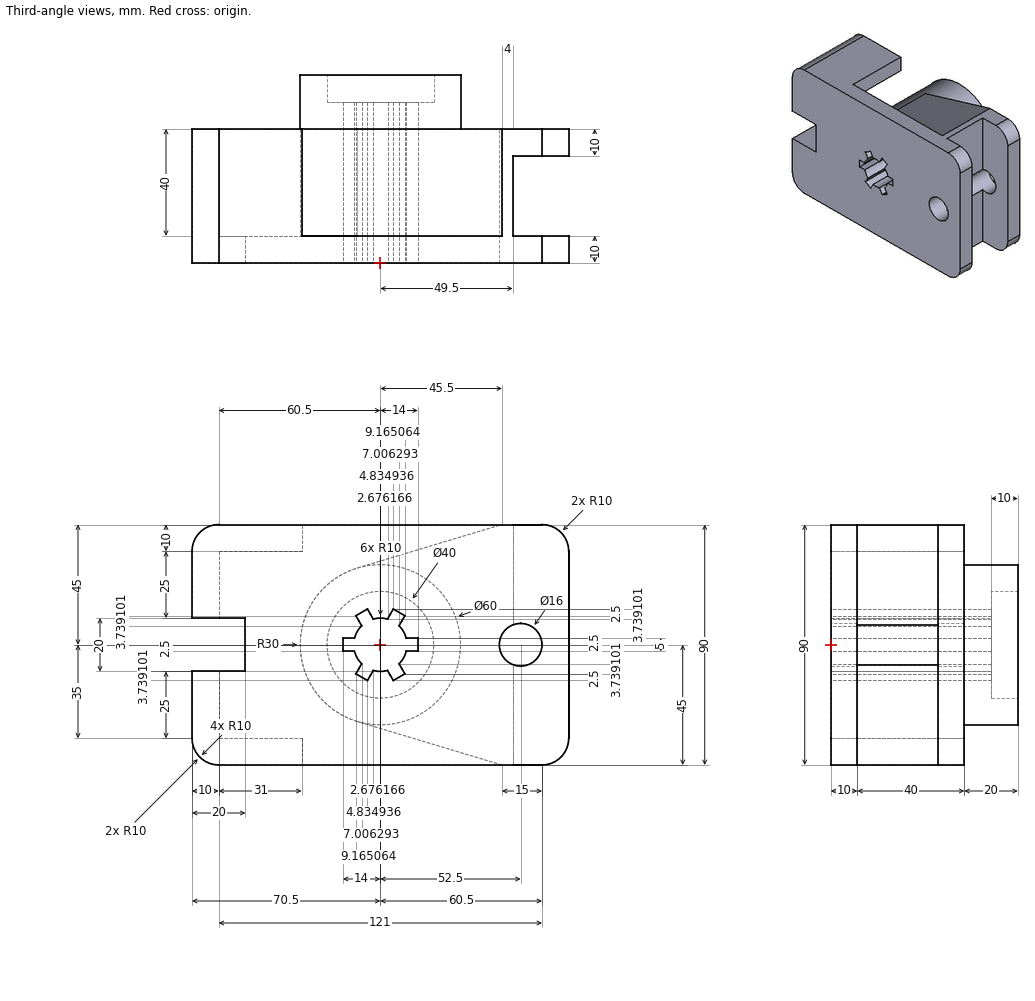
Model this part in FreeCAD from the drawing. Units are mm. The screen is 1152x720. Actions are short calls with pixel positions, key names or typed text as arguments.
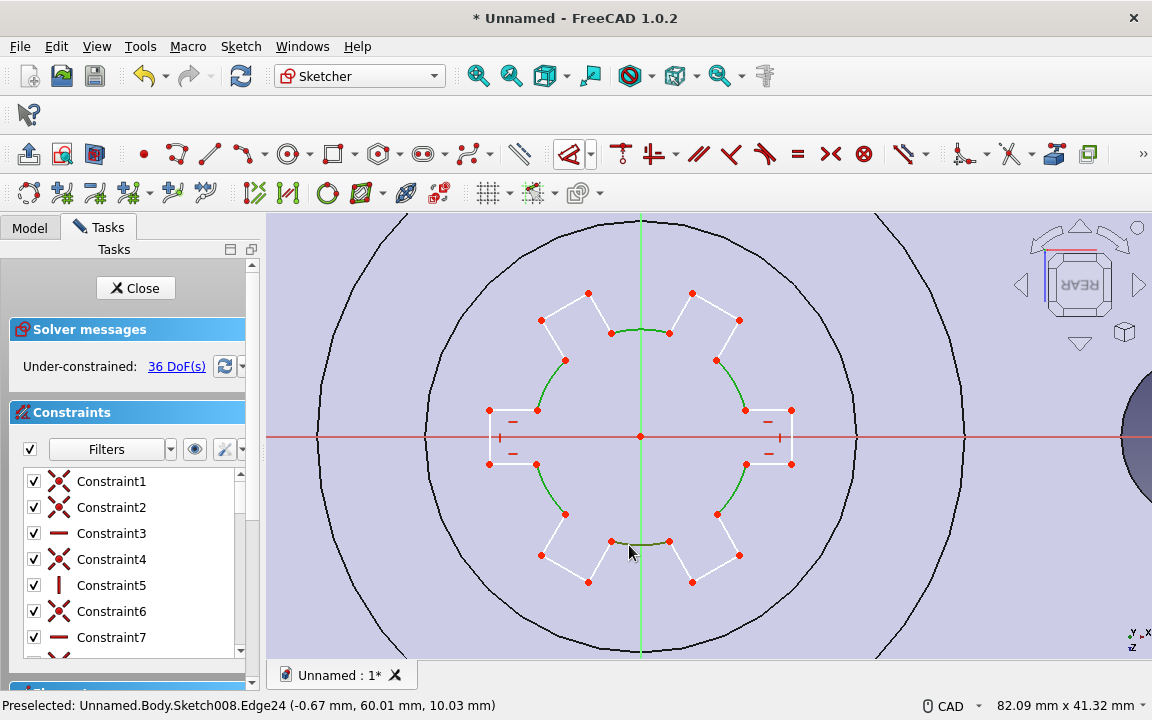
click(798, 154)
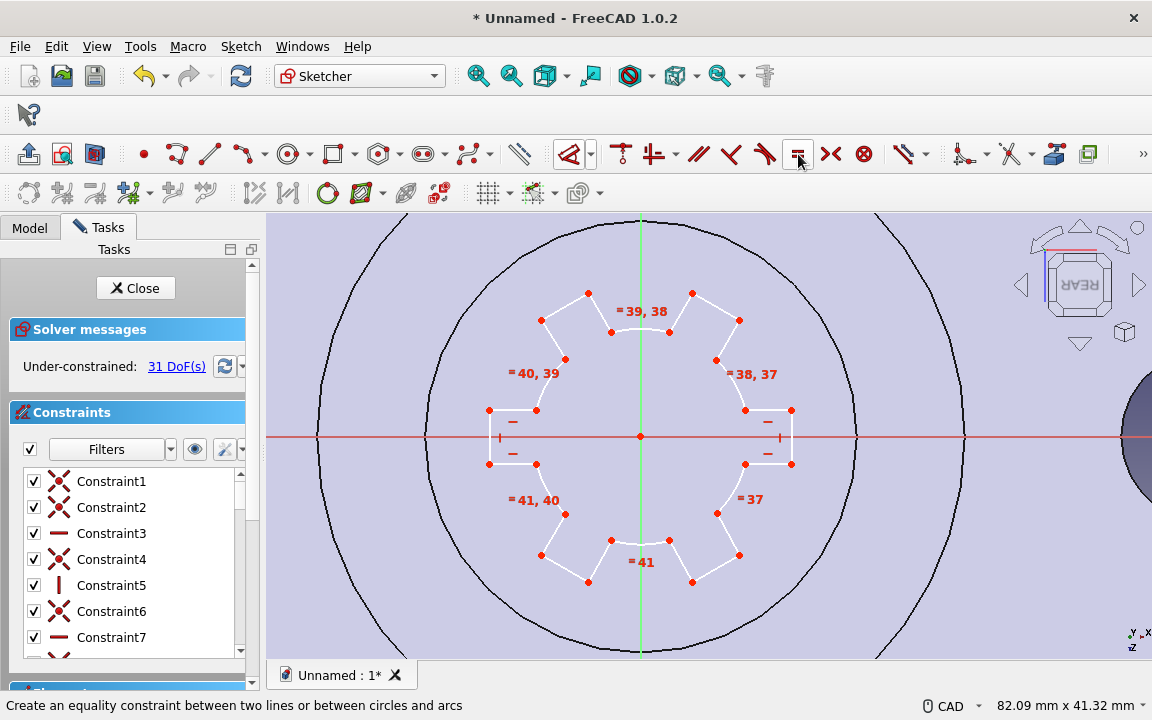
click(728, 500)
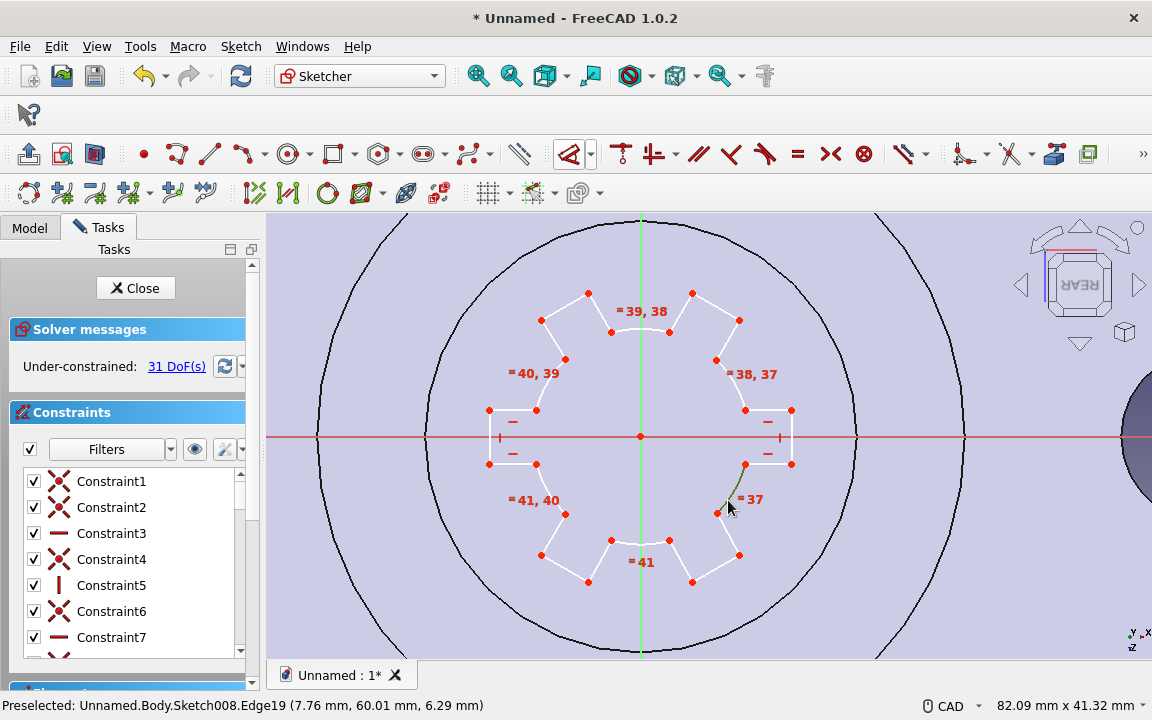
click(590, 154)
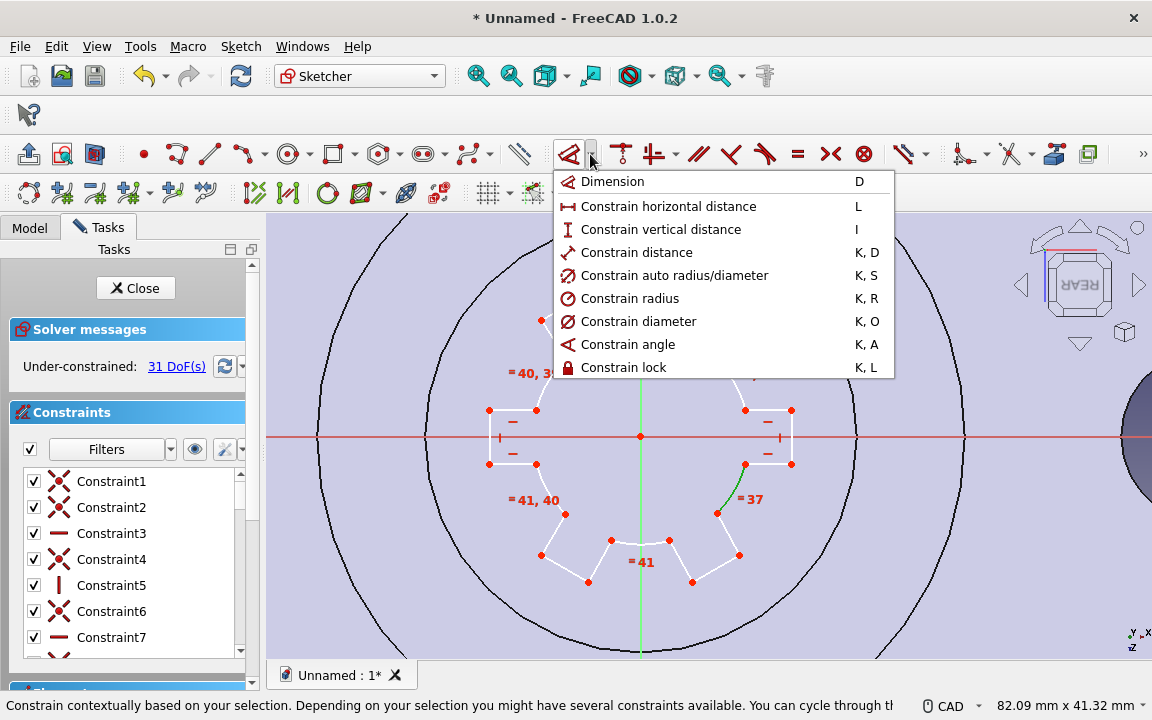
click(724, 298)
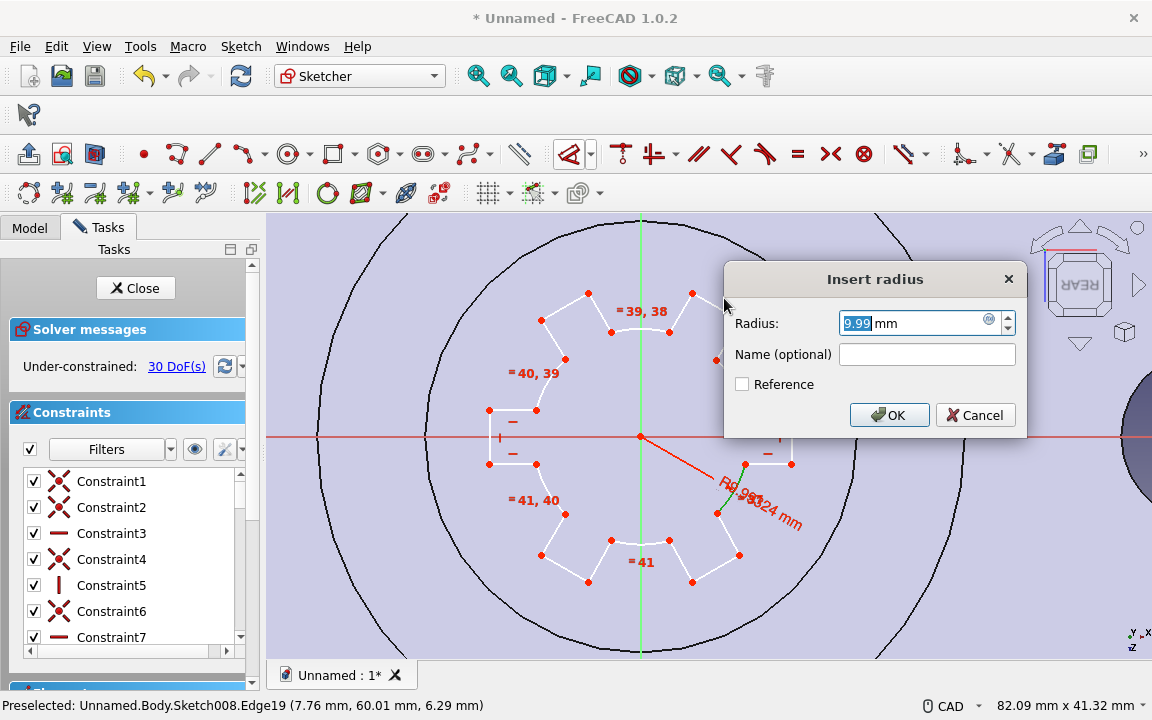
text(10)
key(Return)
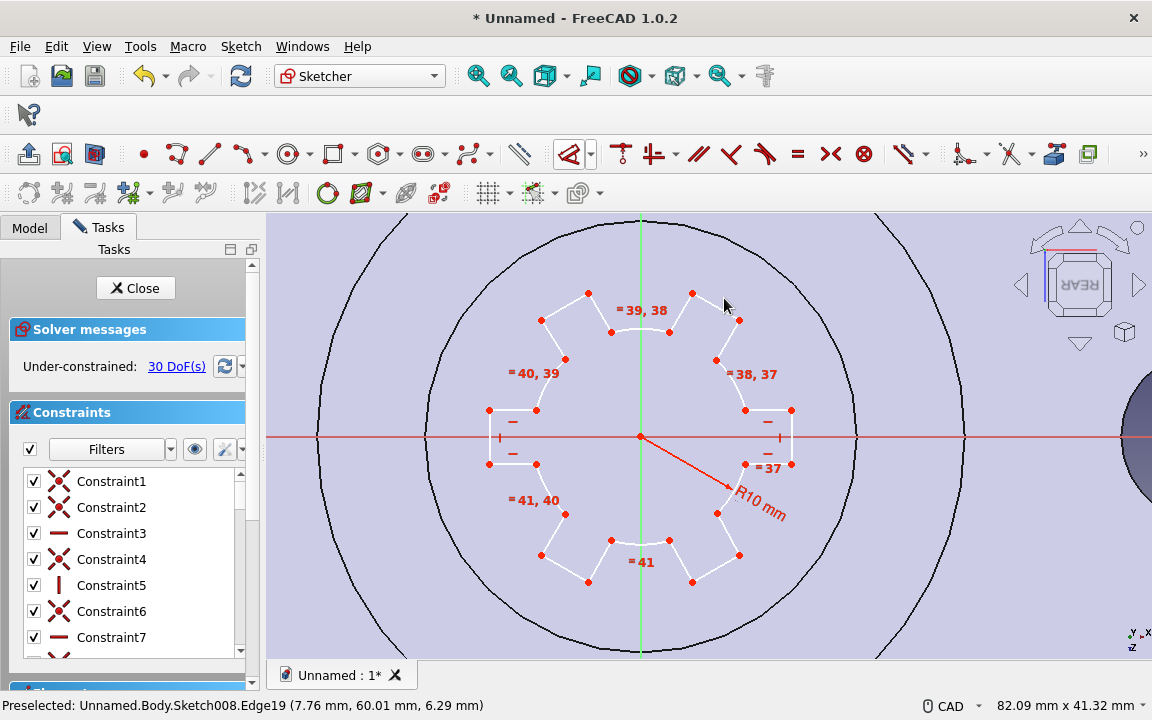
click(792, 448)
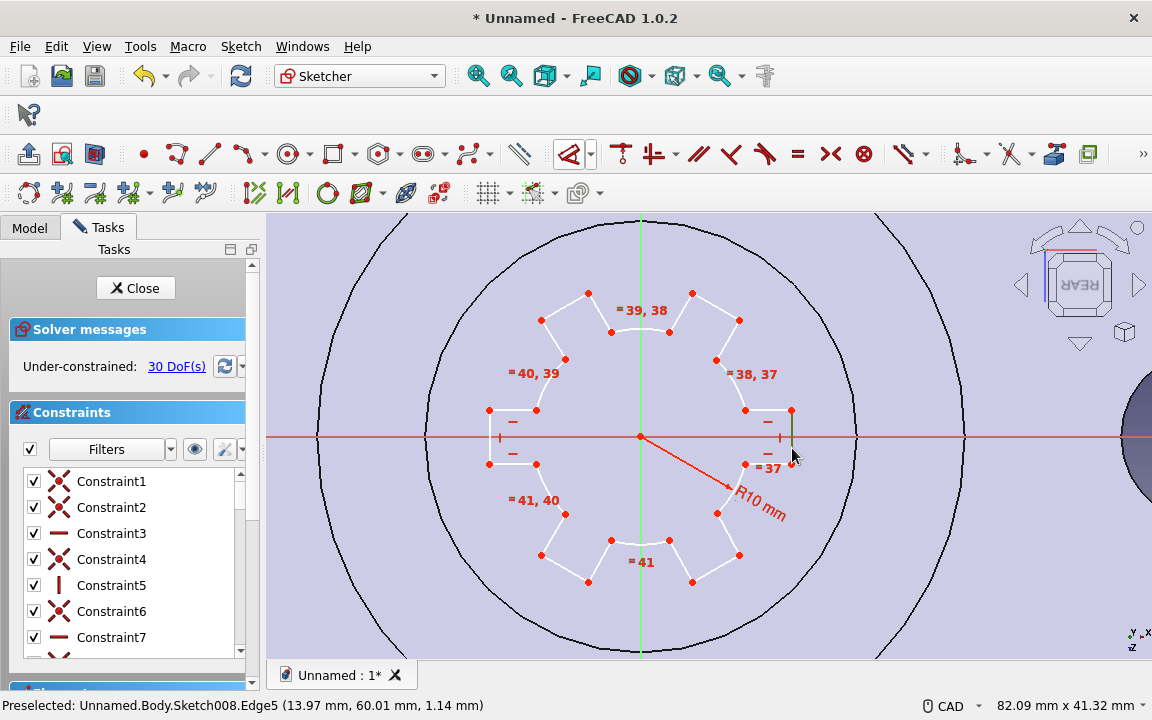
key(i)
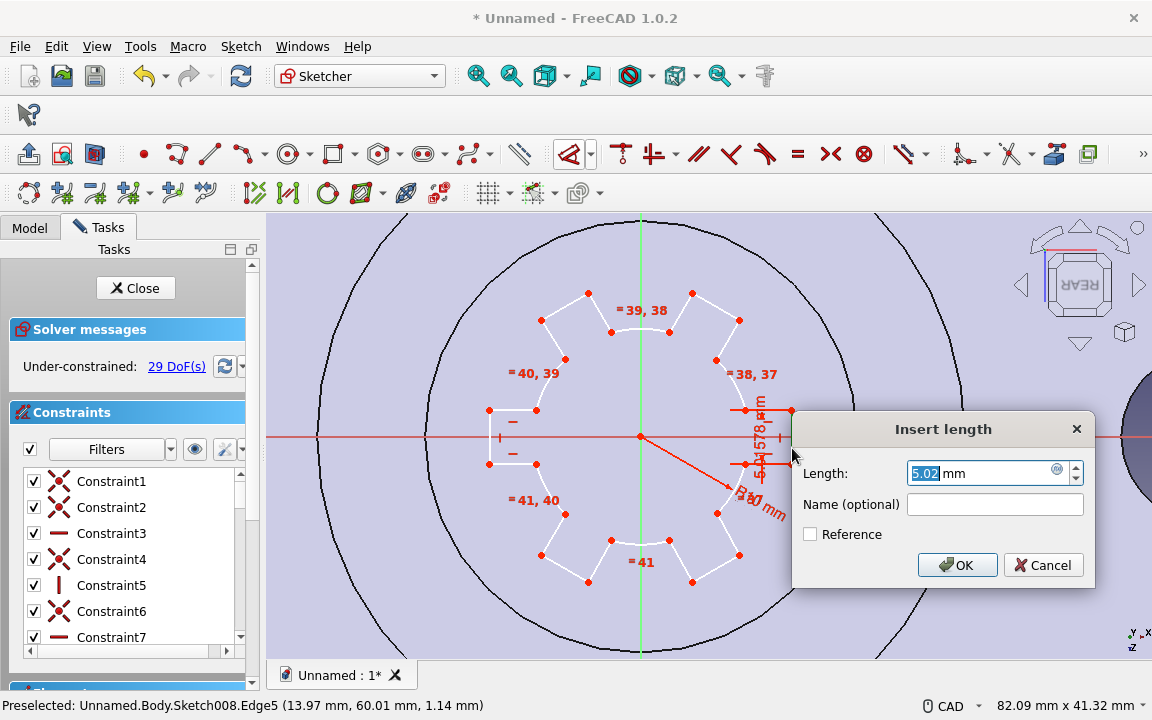
text(5)
key(Return)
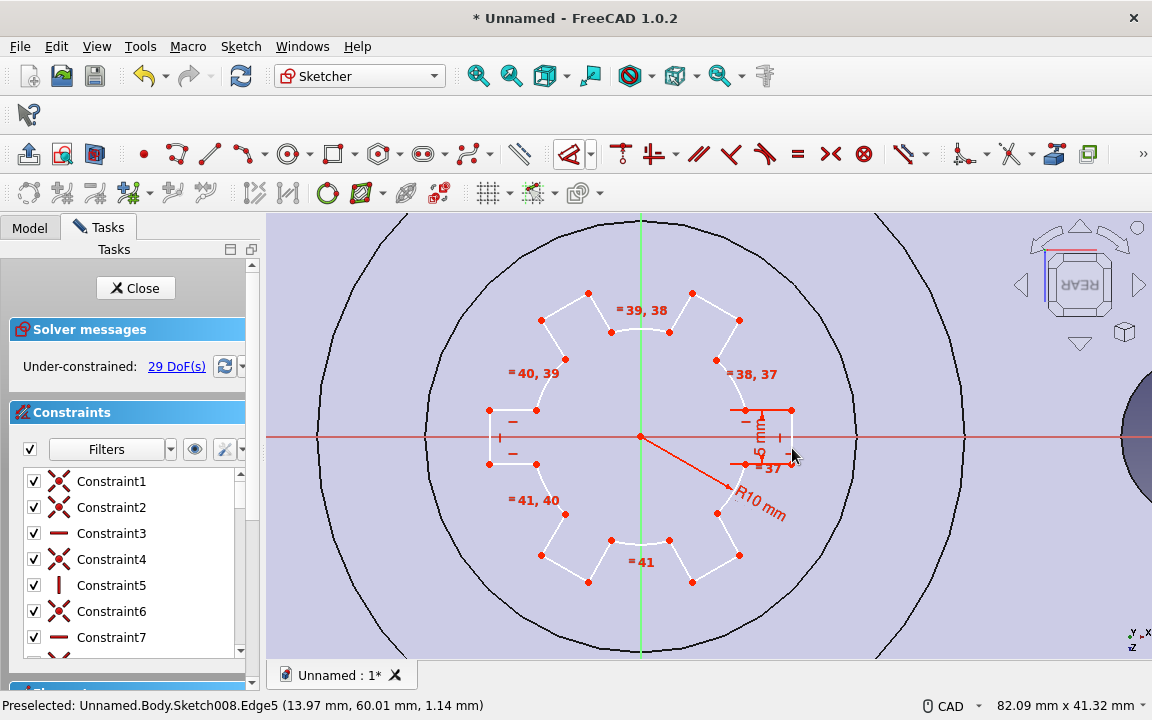
scroll(490, 426, up, 2)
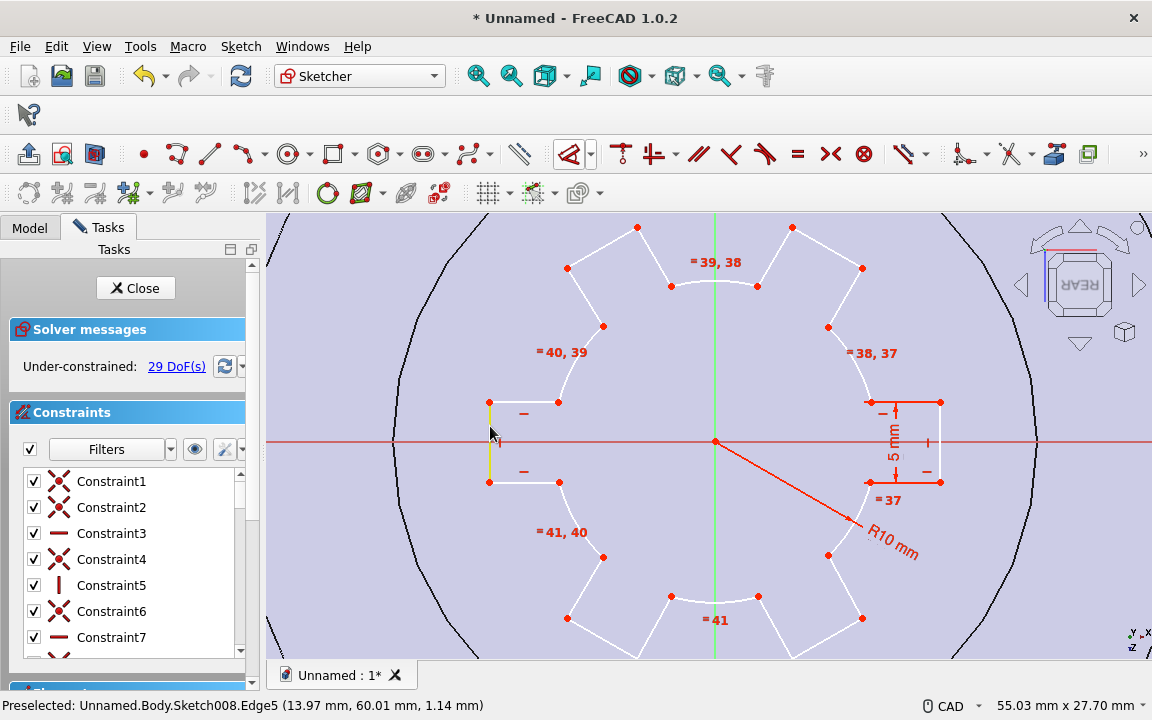
click(490, 426)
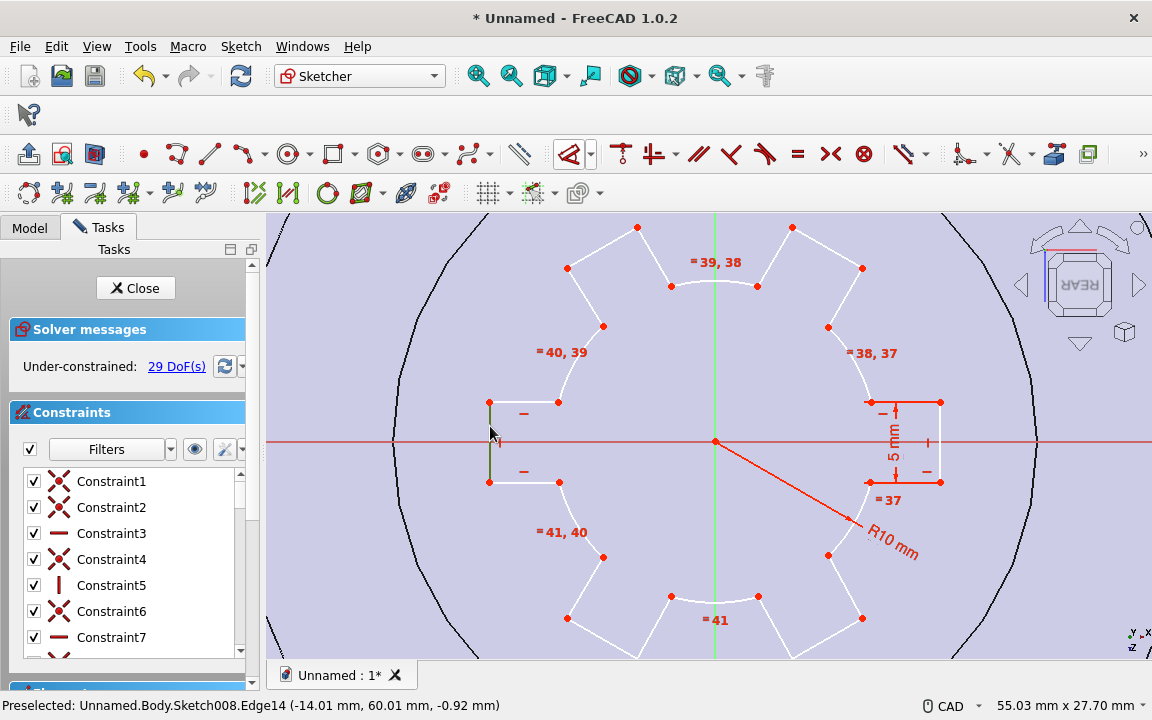
key(i)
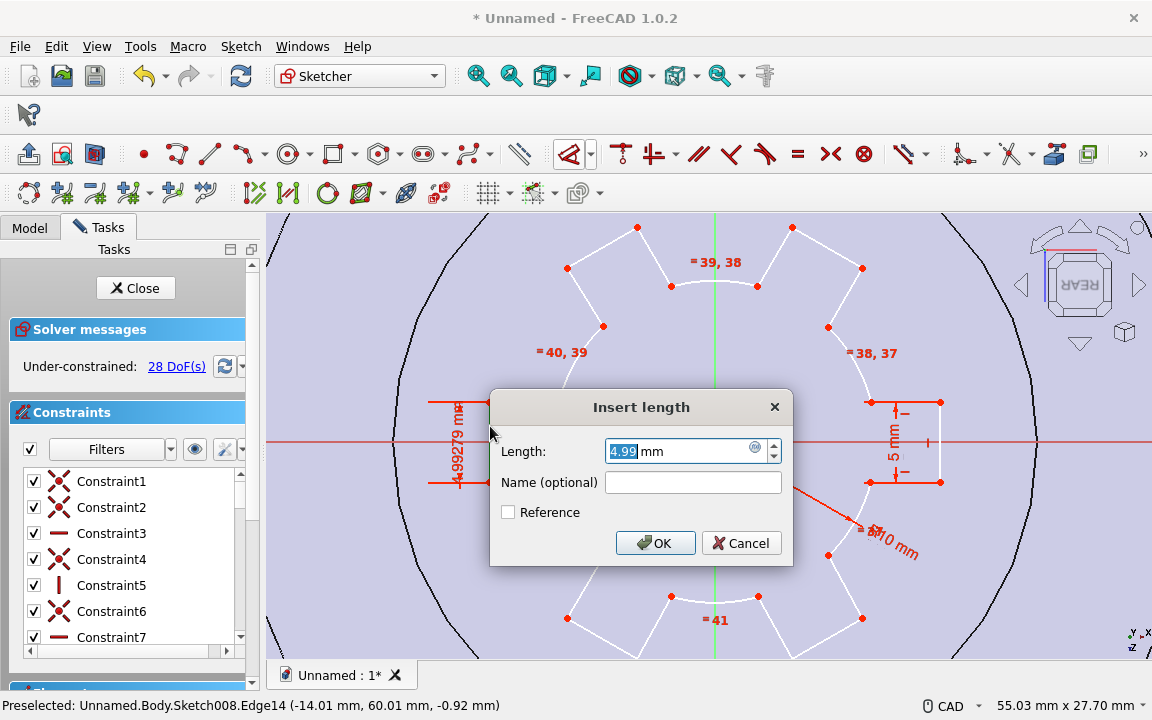
text(5)
key(Return)